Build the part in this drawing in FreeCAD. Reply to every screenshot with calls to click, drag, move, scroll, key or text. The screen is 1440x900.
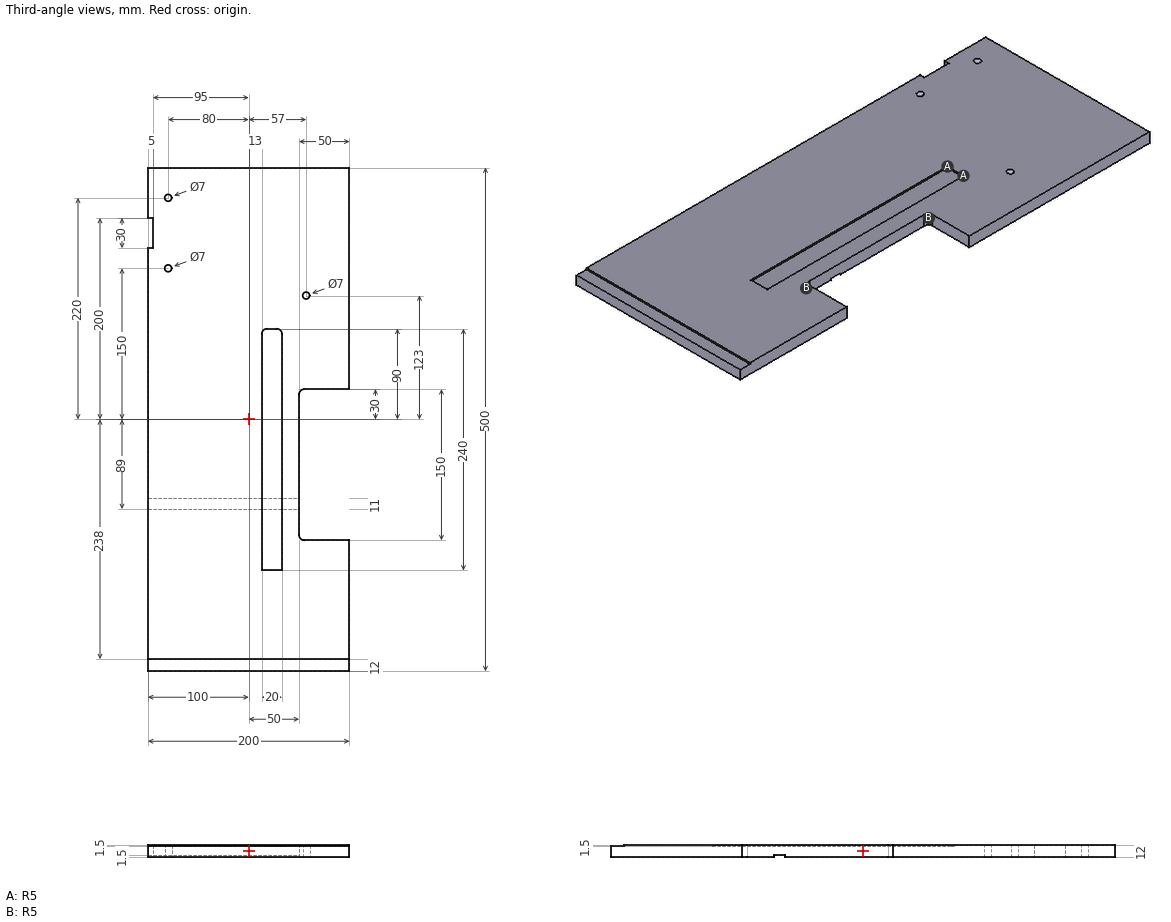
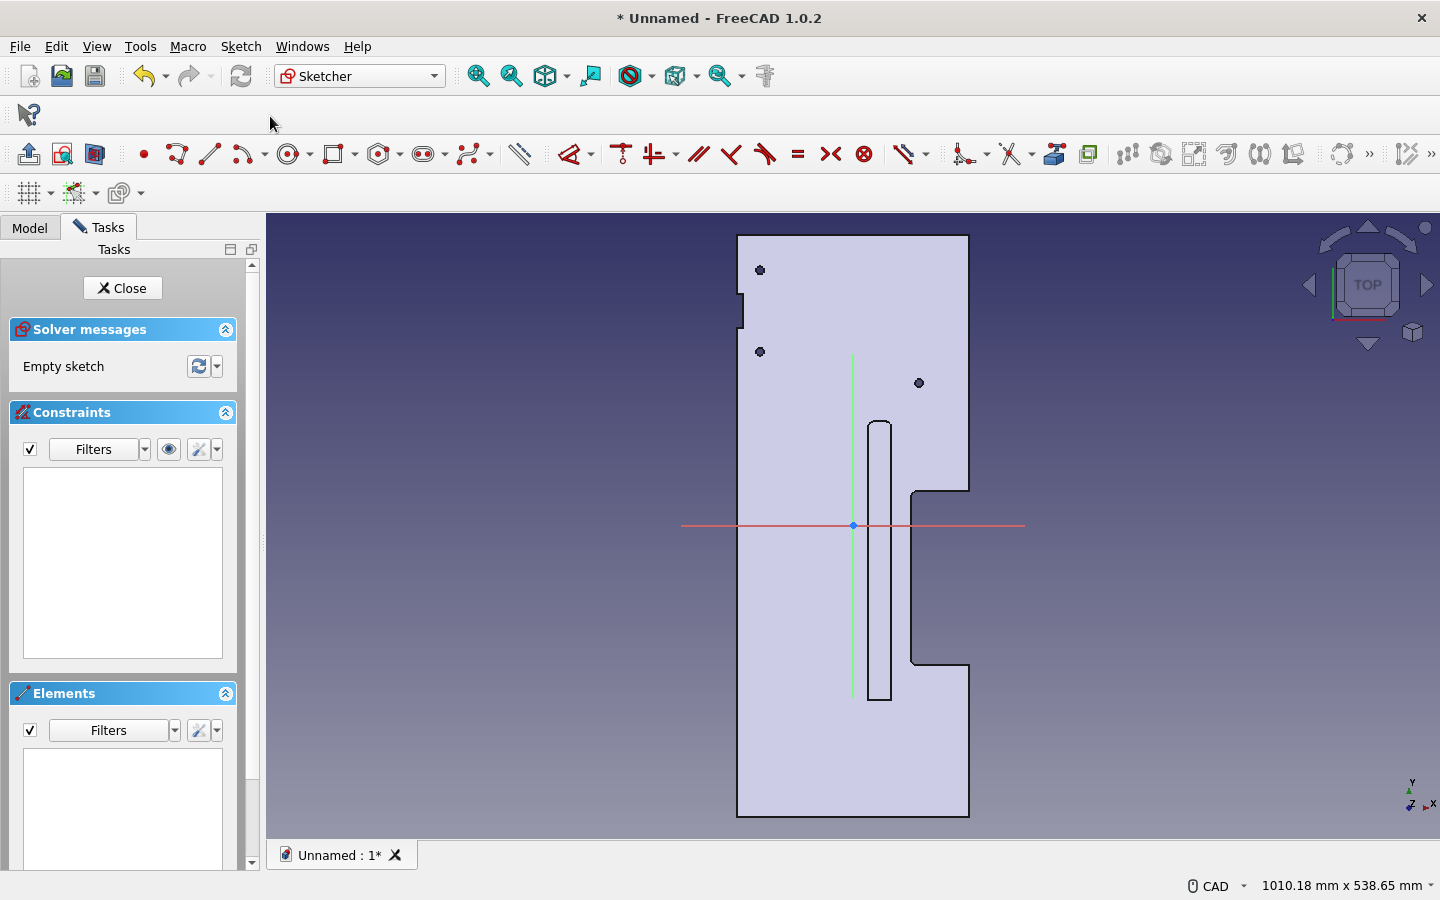
scroll(475, 241, down, 1)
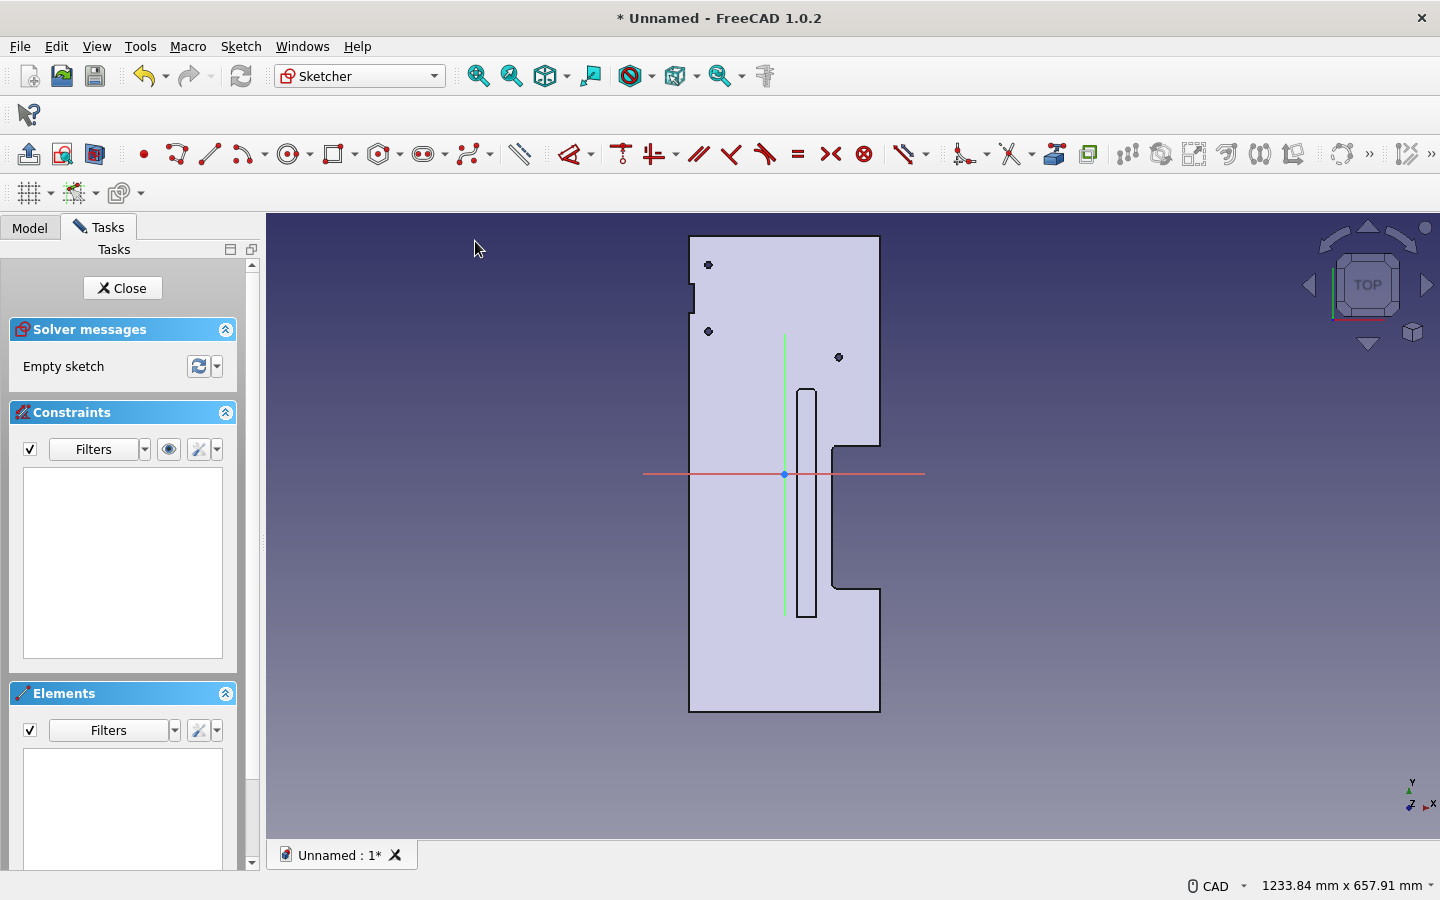
scroll(785, 675, up, 3)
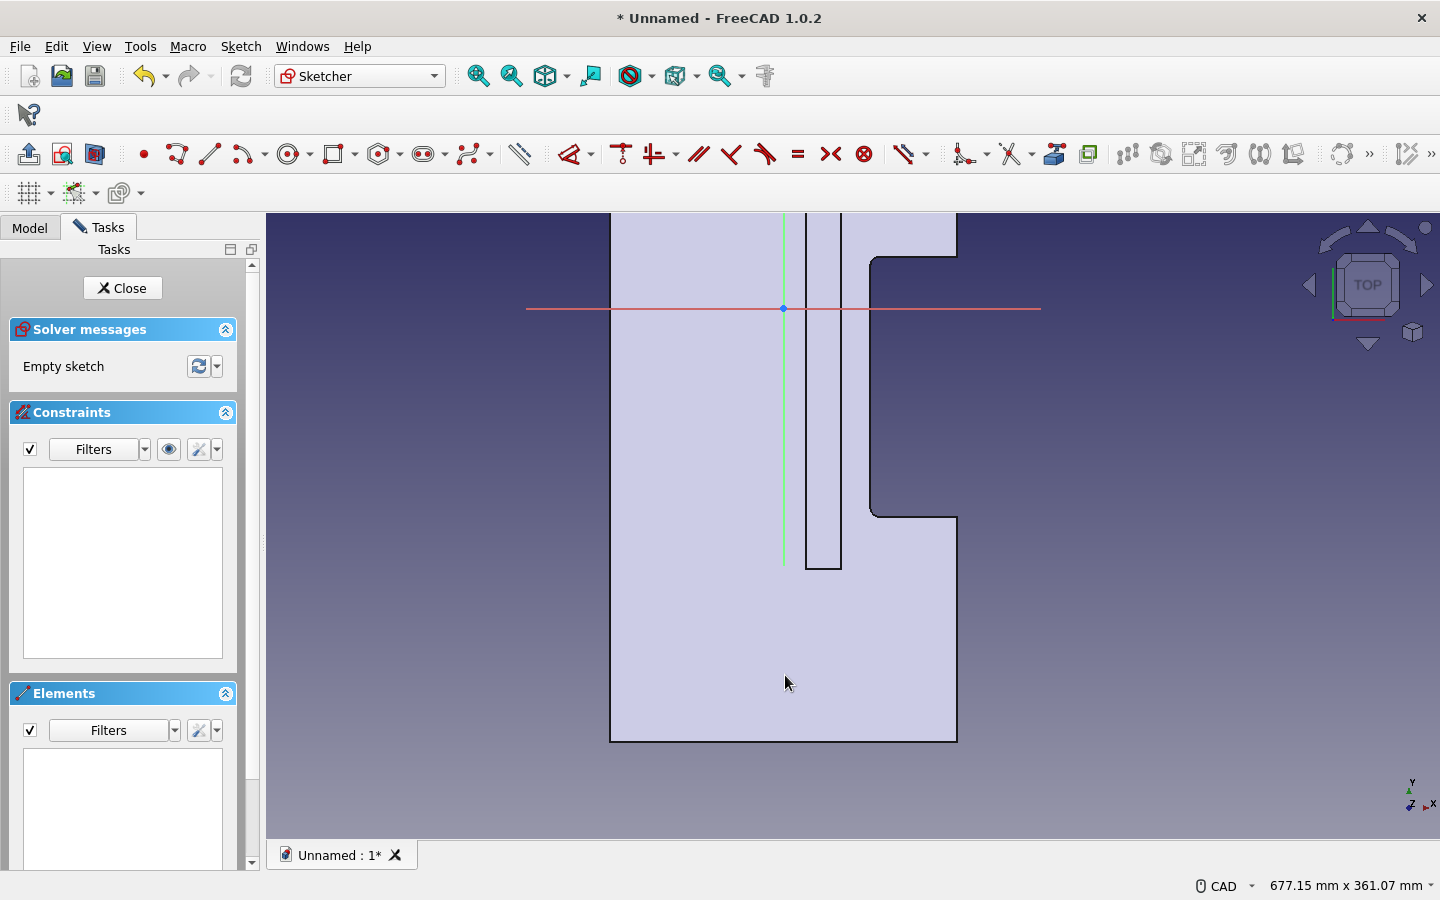
click(332, 154)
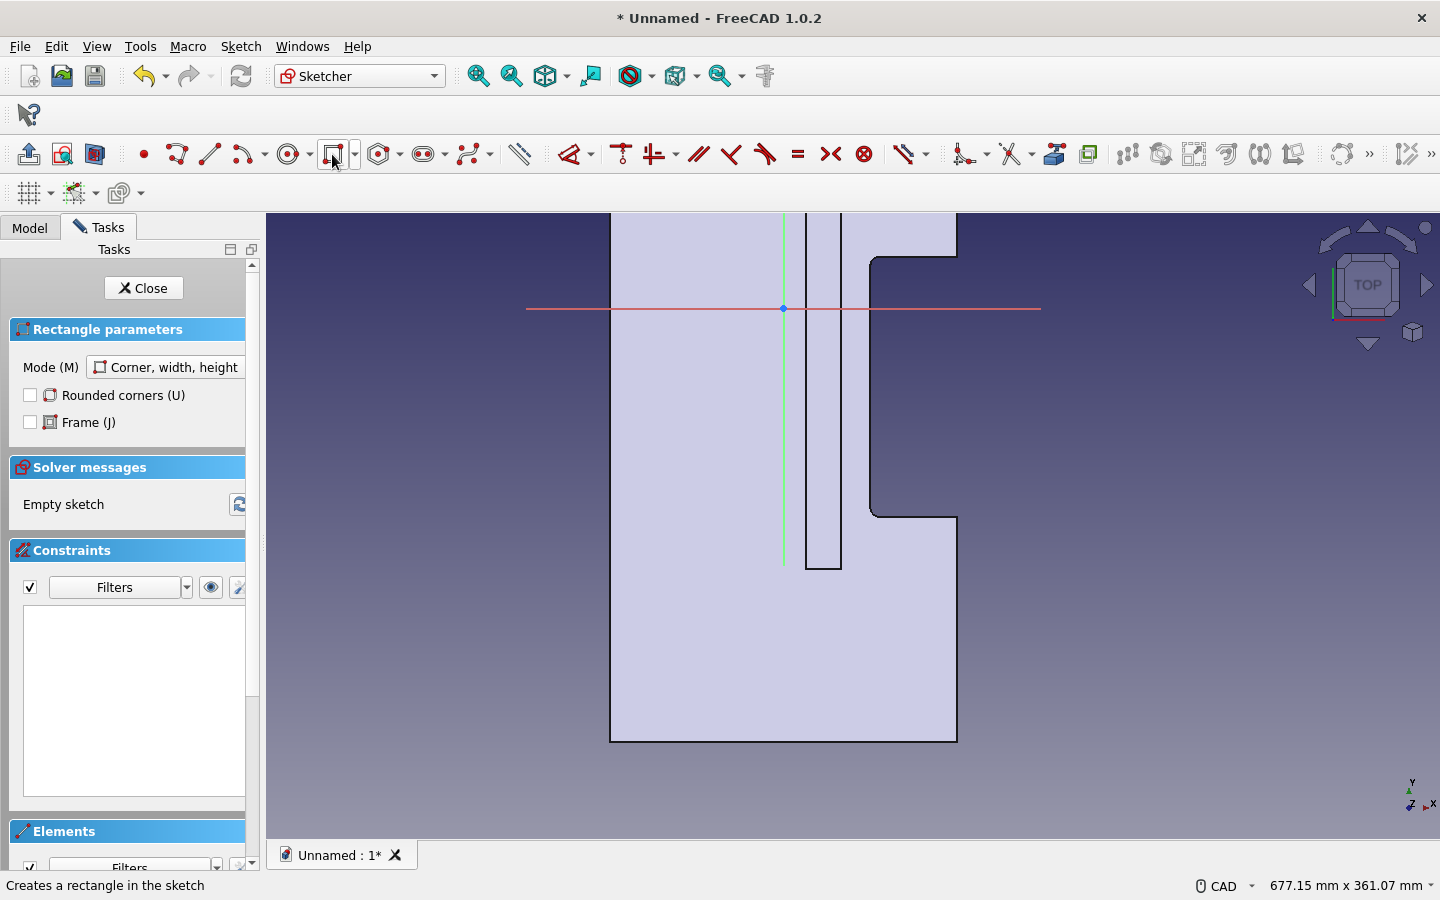
click(610, 721)
move(957, 742)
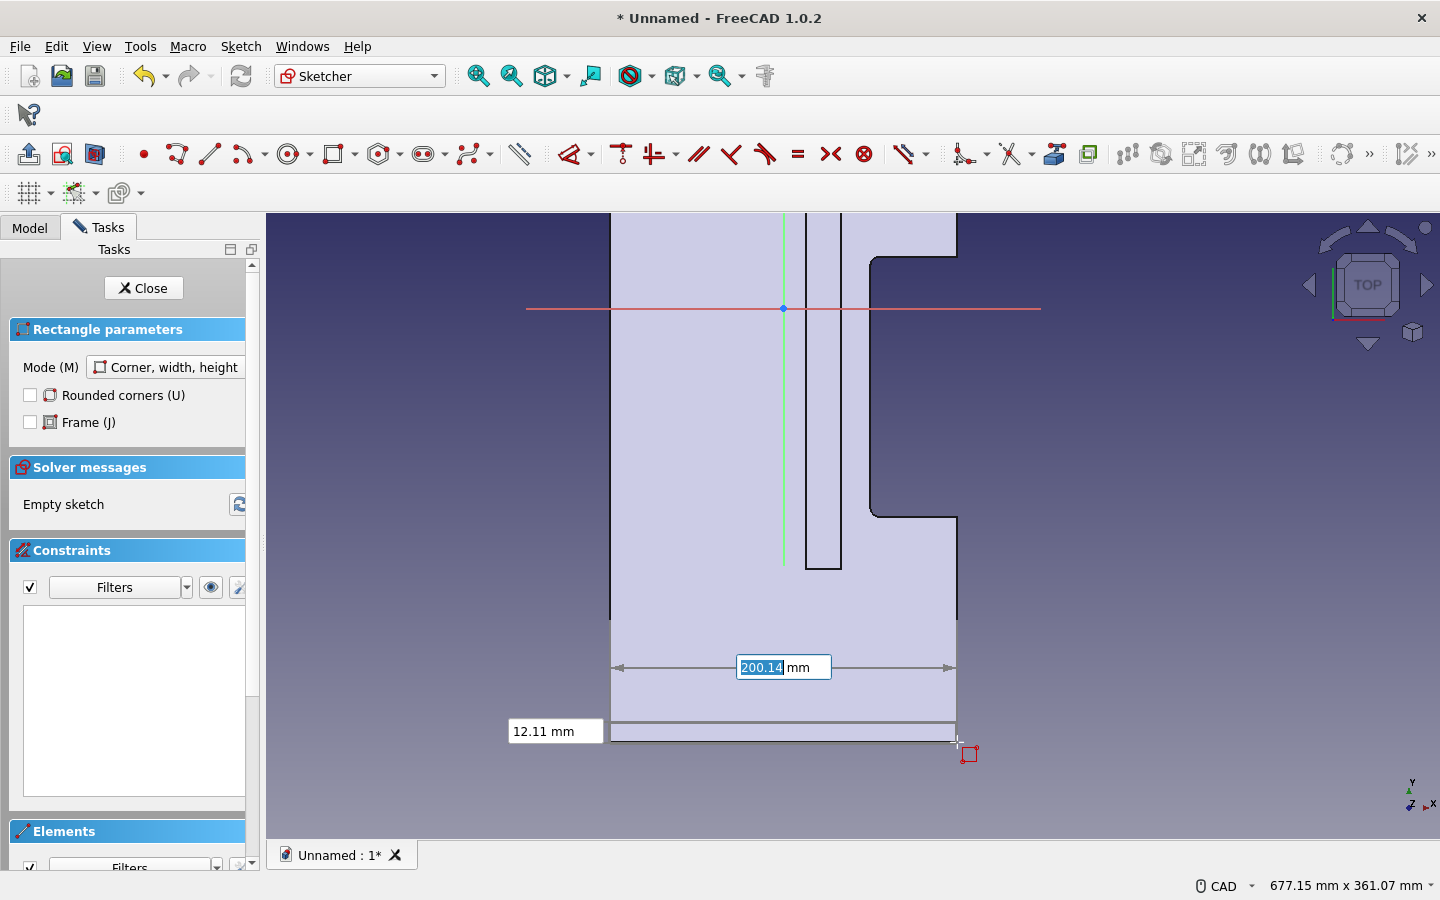
text(200)
key(Tab)
text(12)
key(Return)
key(Escape)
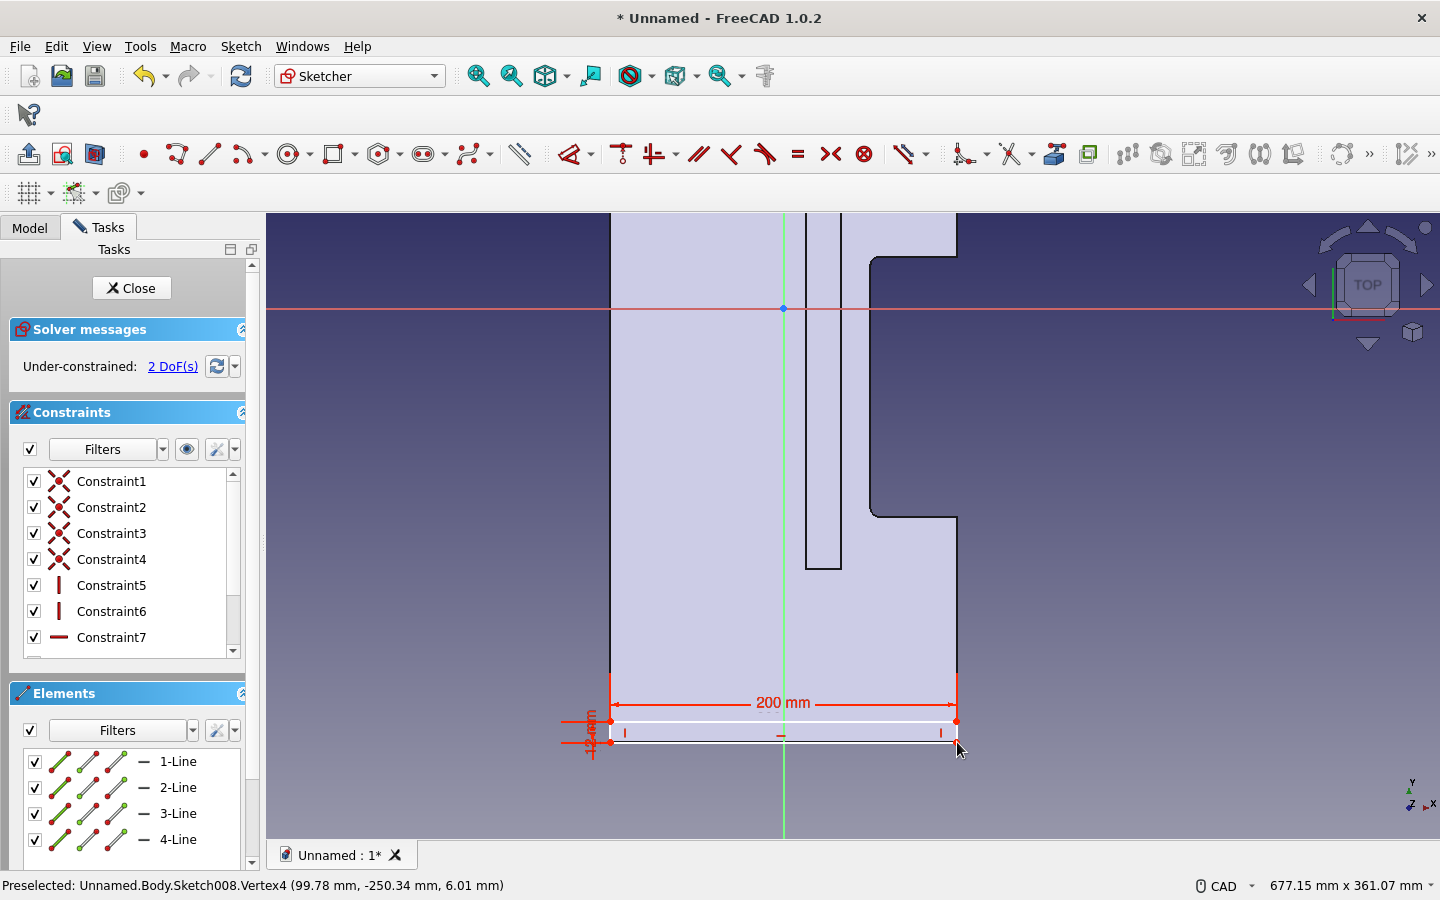
click(568, 154)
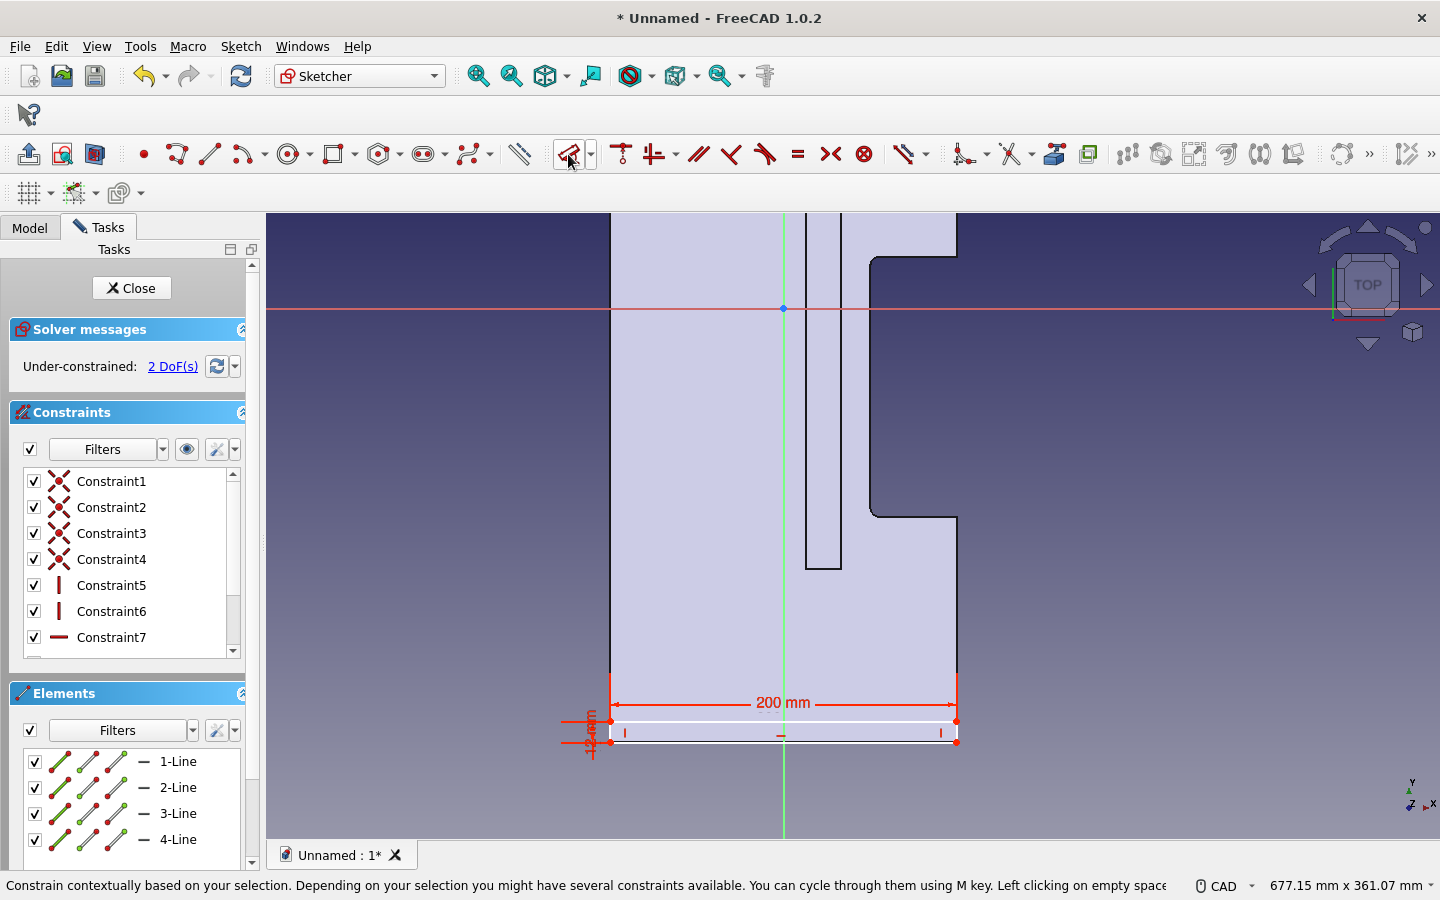
click(610, 722)
click(697, 275)